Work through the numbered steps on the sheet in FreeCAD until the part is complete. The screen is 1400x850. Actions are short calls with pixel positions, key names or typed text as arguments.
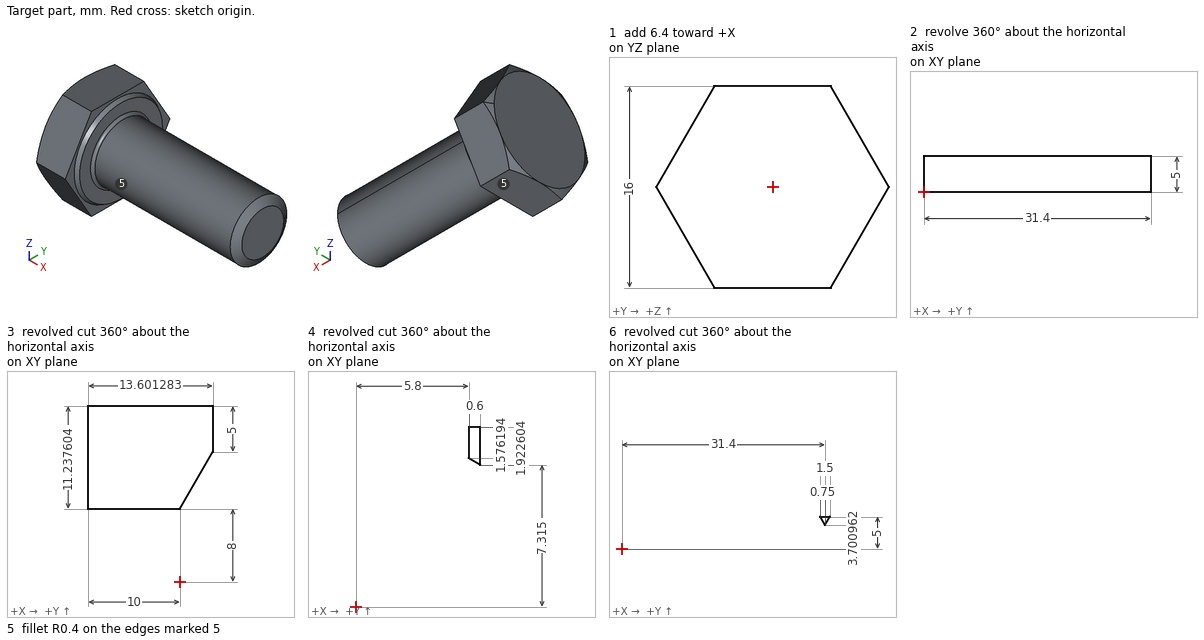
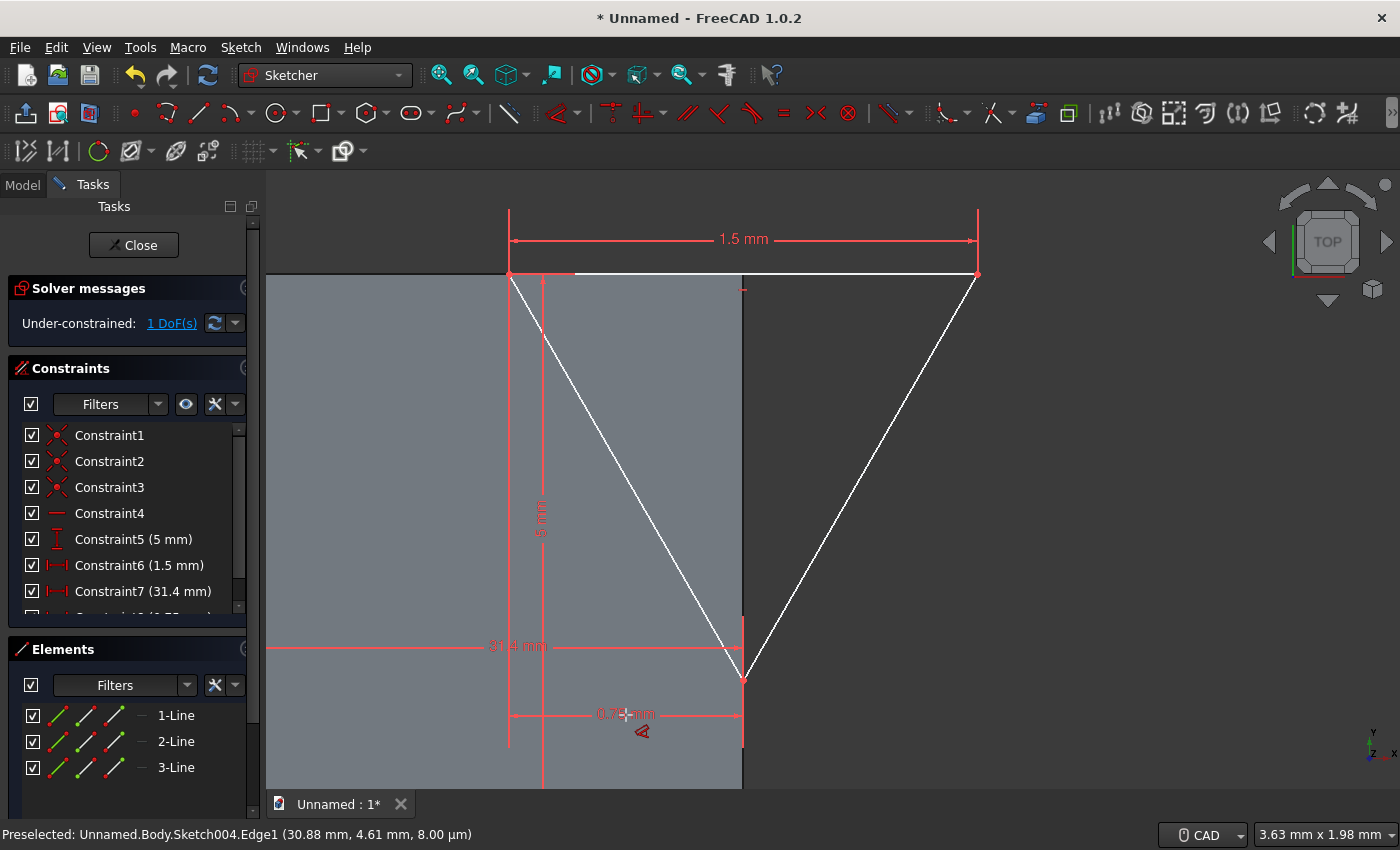
click(743, 681)
click(777, 721)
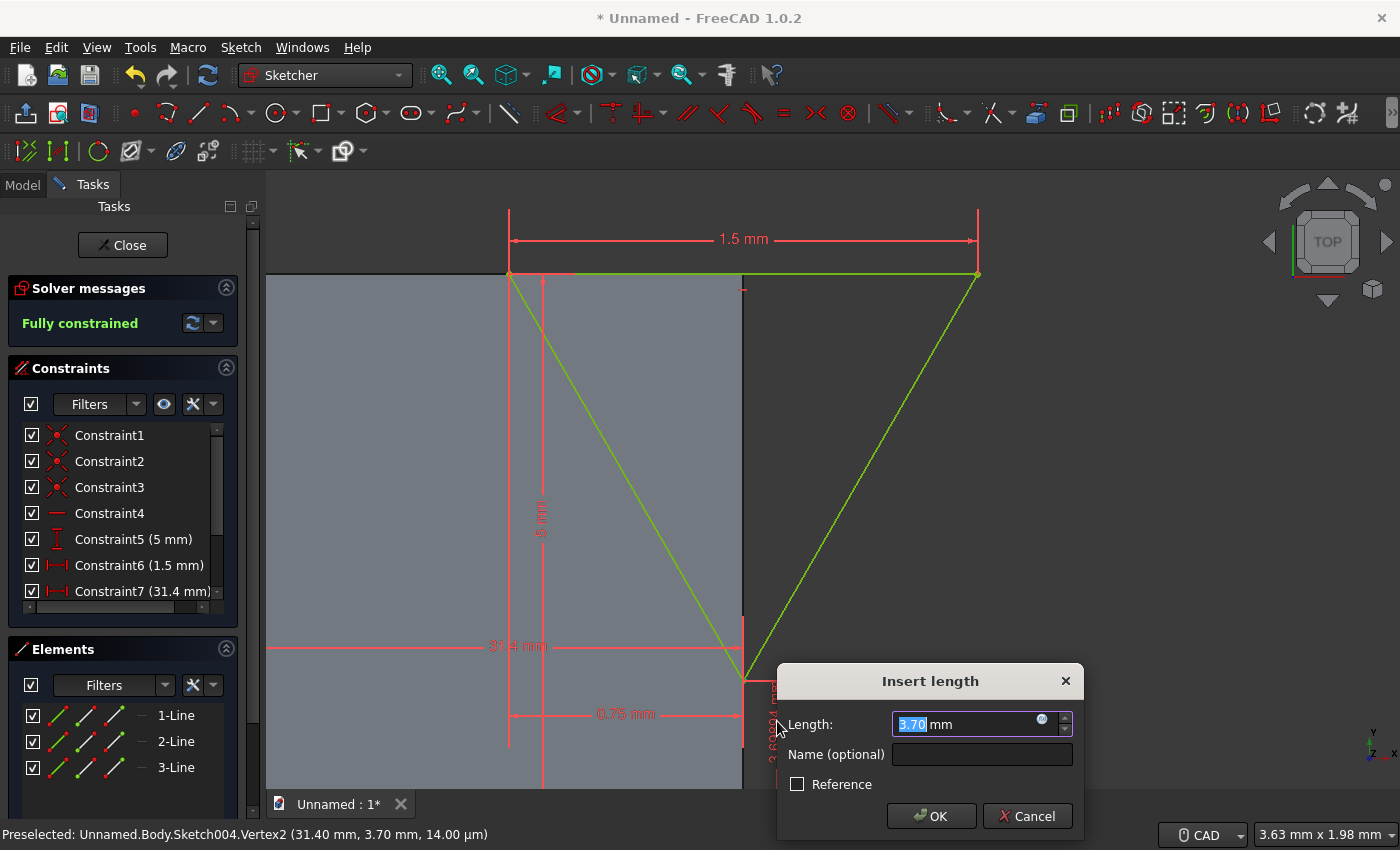
text(3.700962)
key(Return)
key(Escape)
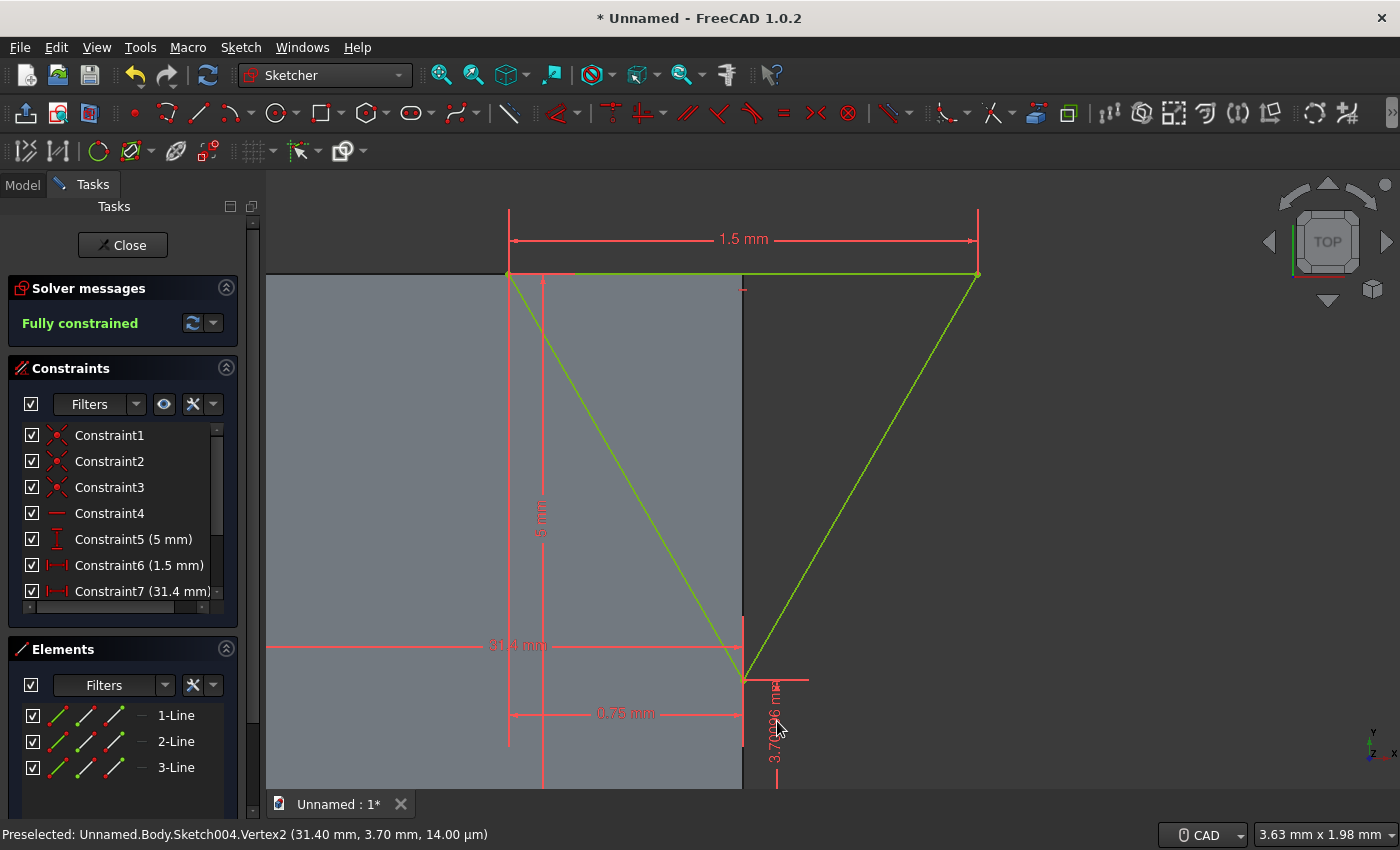
click(123, 245)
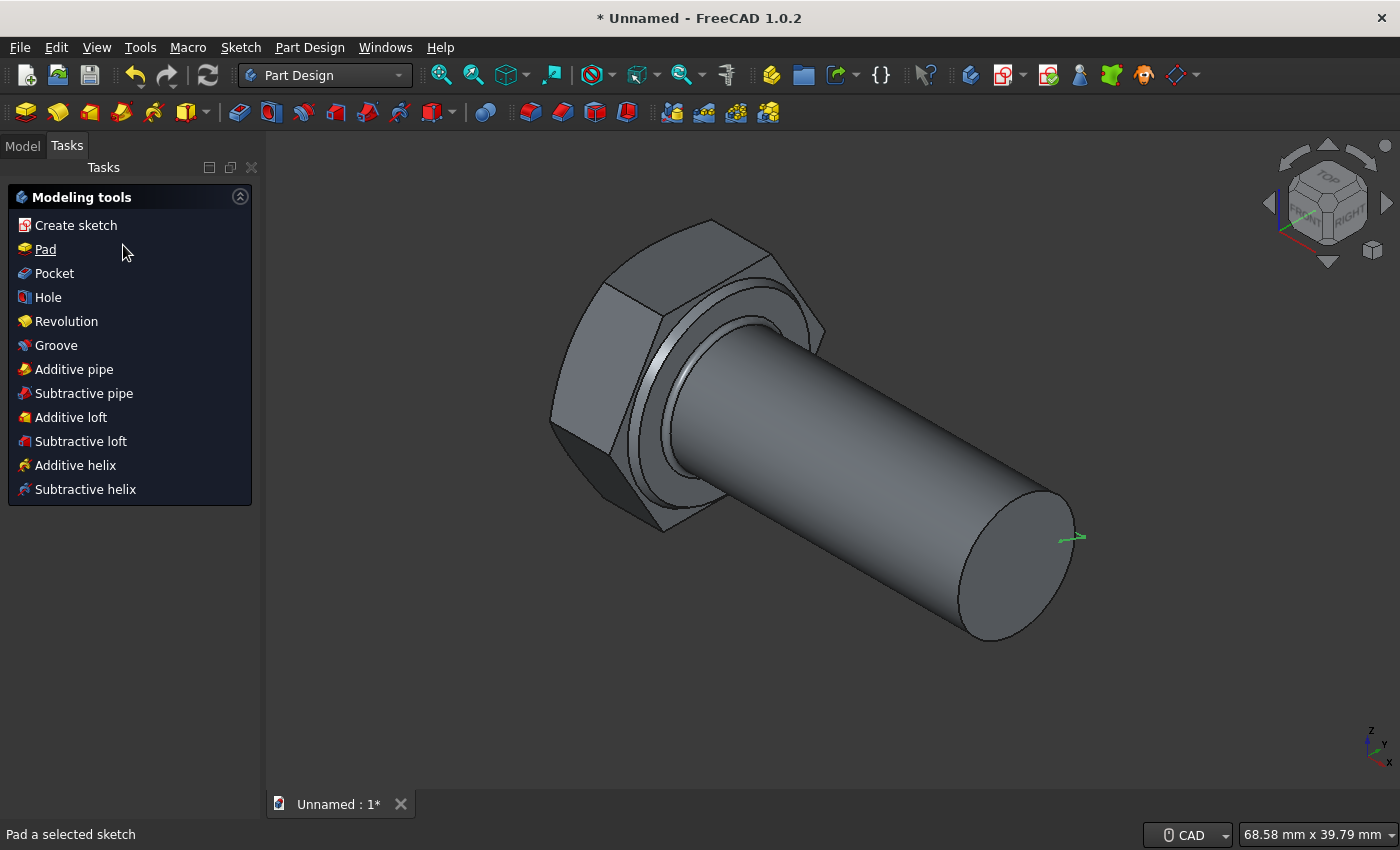
click(304, 112)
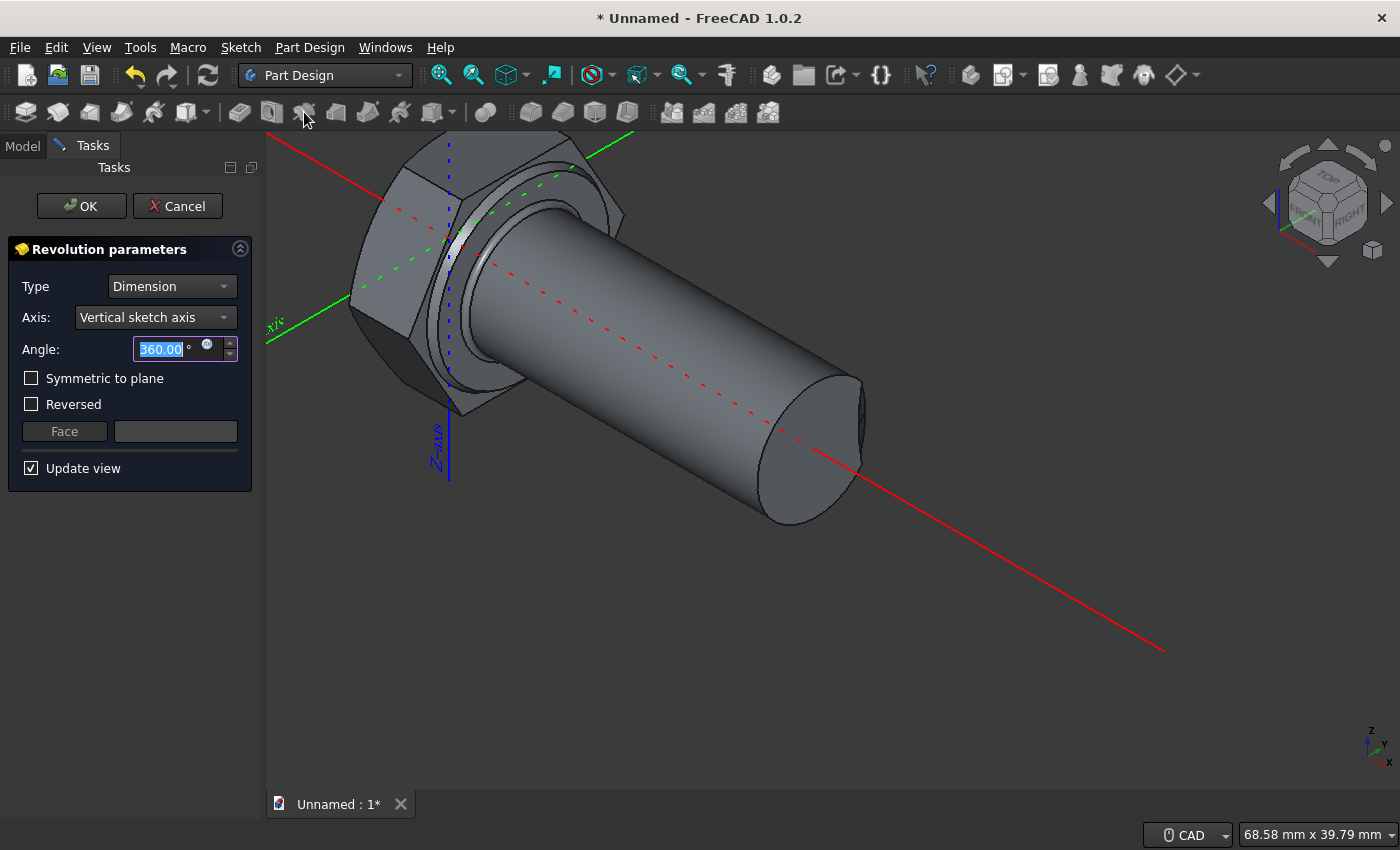
click(156, 318)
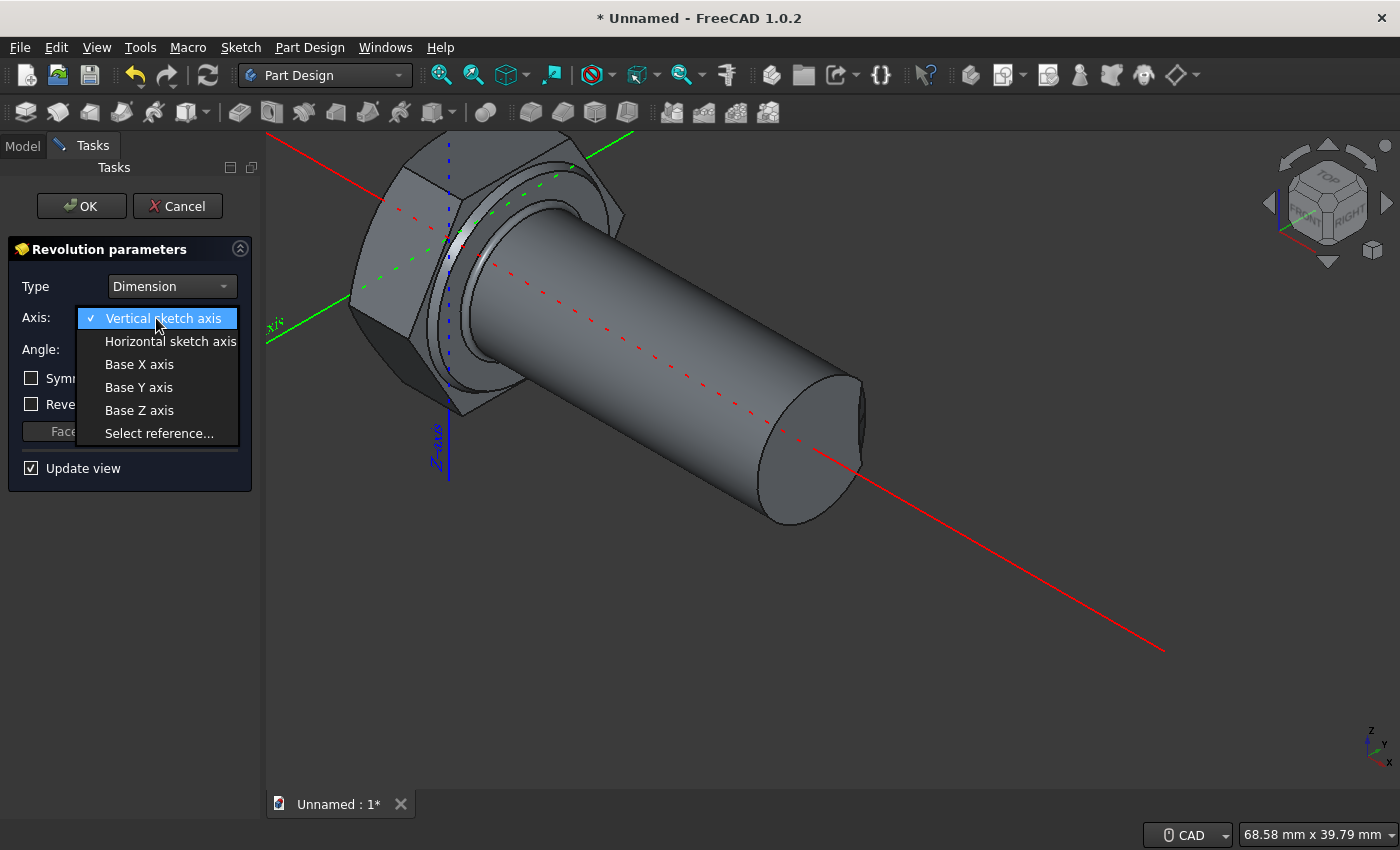
click(156, 342)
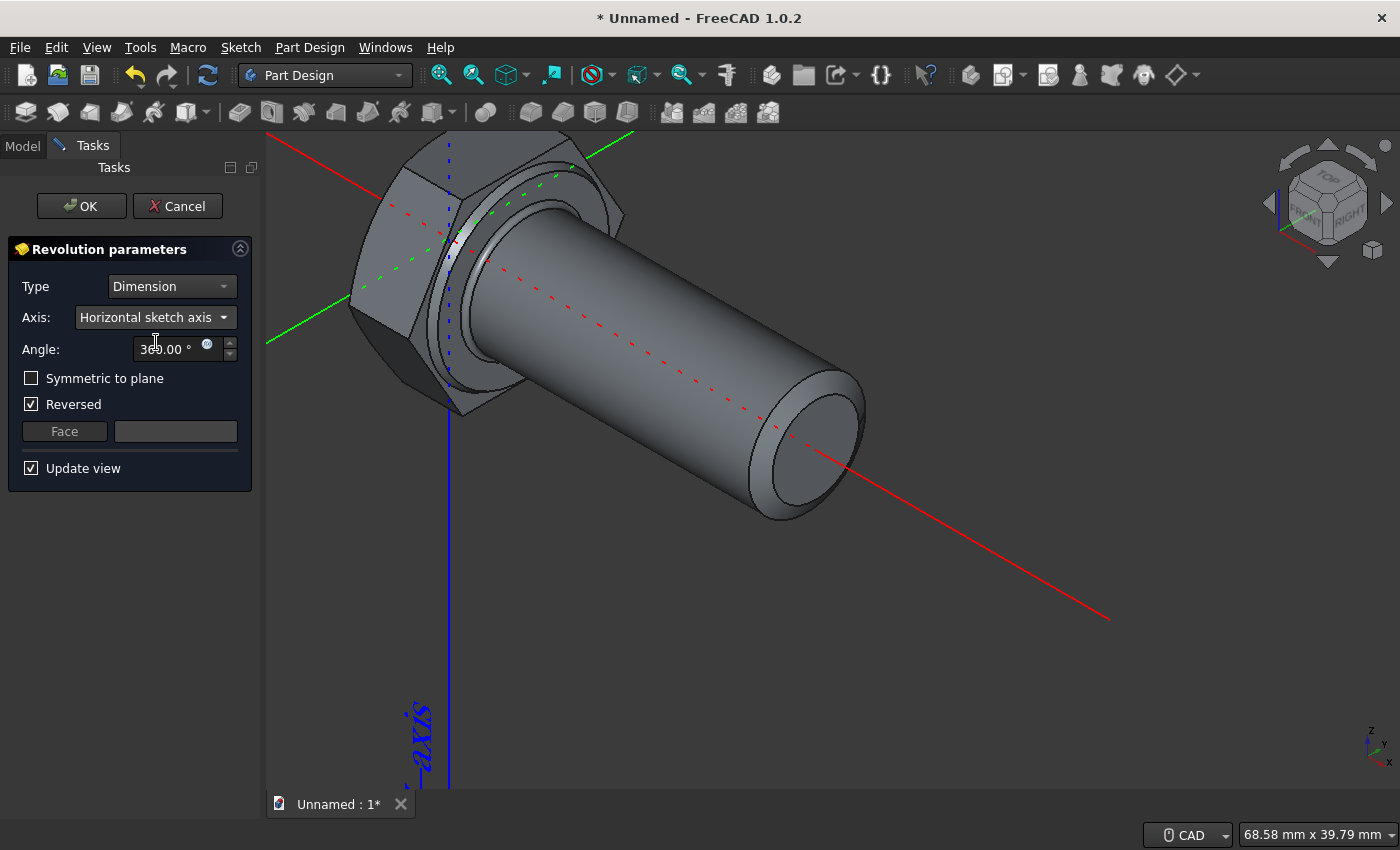
click(82, 206)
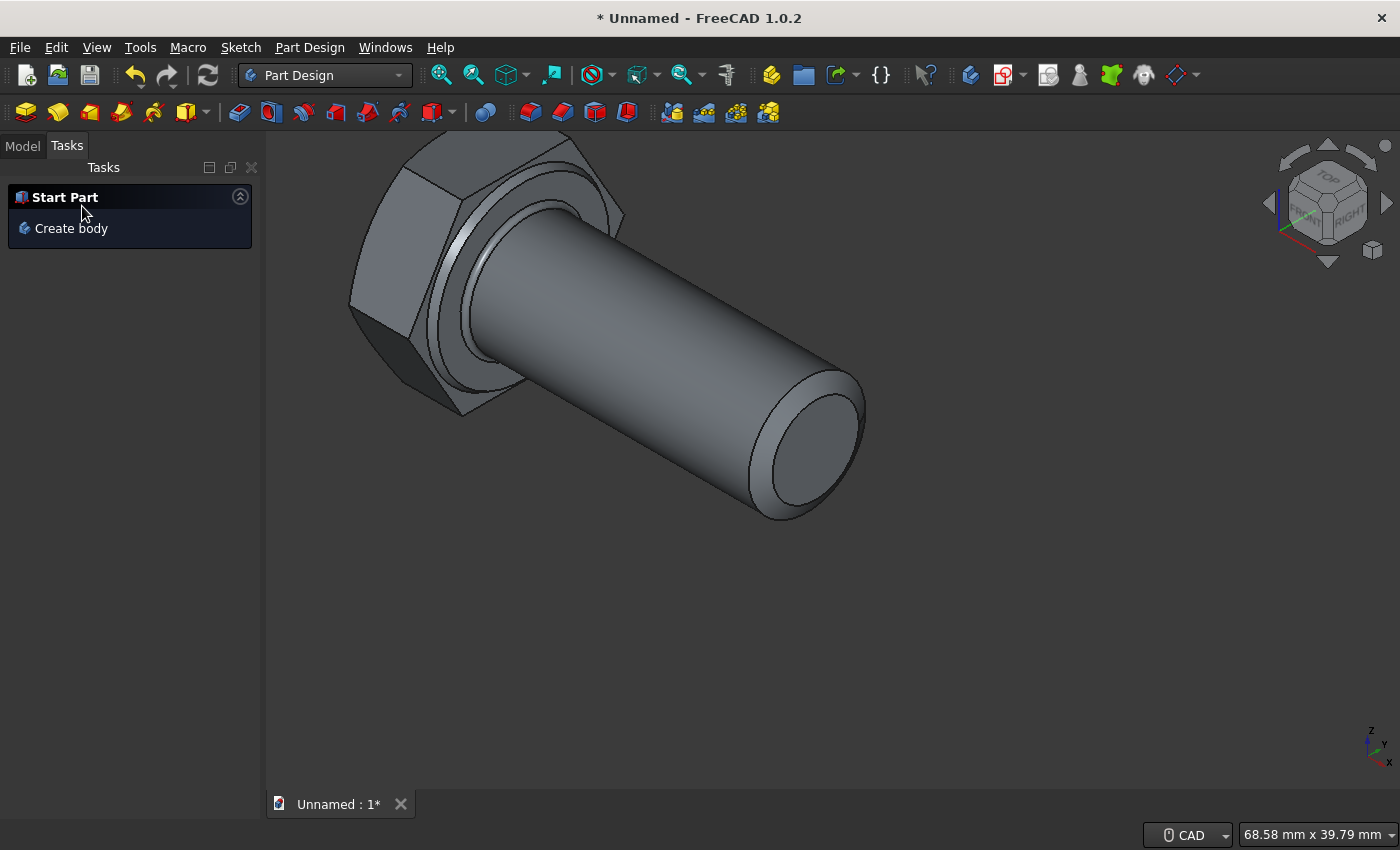
click(442, 76)